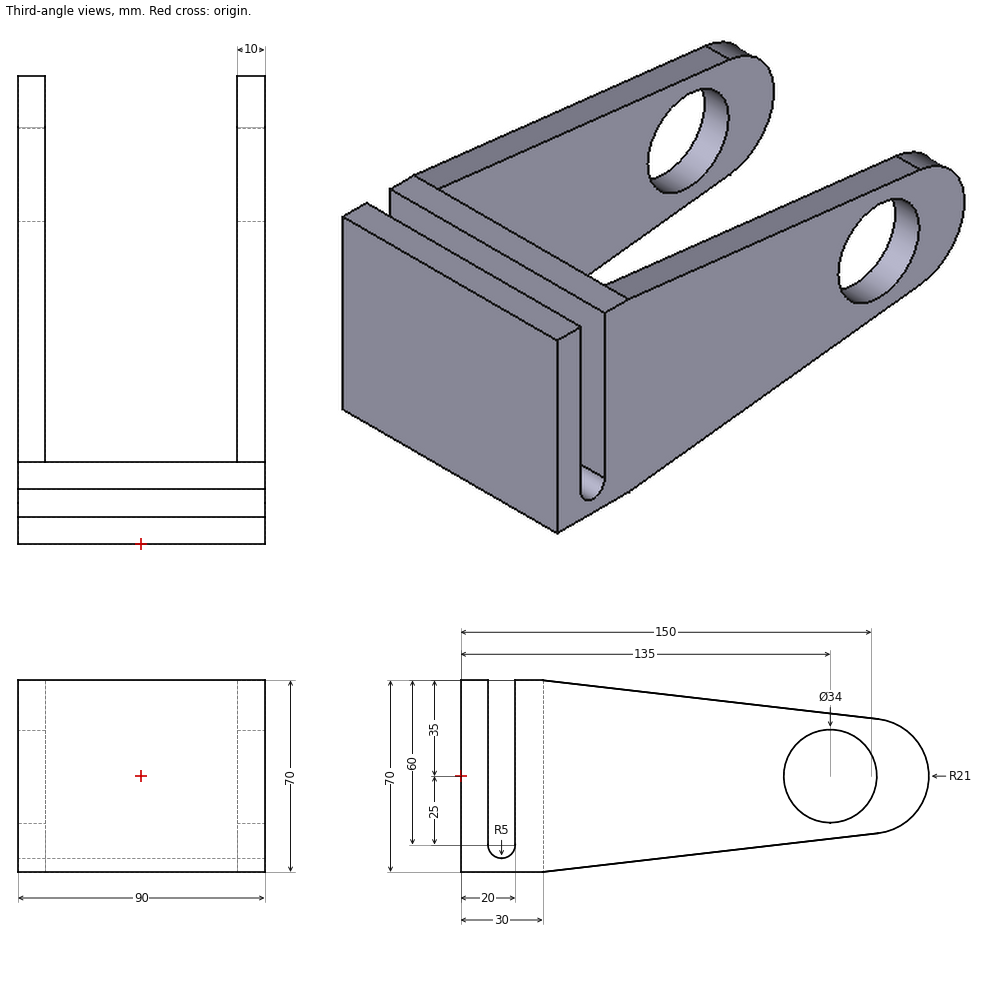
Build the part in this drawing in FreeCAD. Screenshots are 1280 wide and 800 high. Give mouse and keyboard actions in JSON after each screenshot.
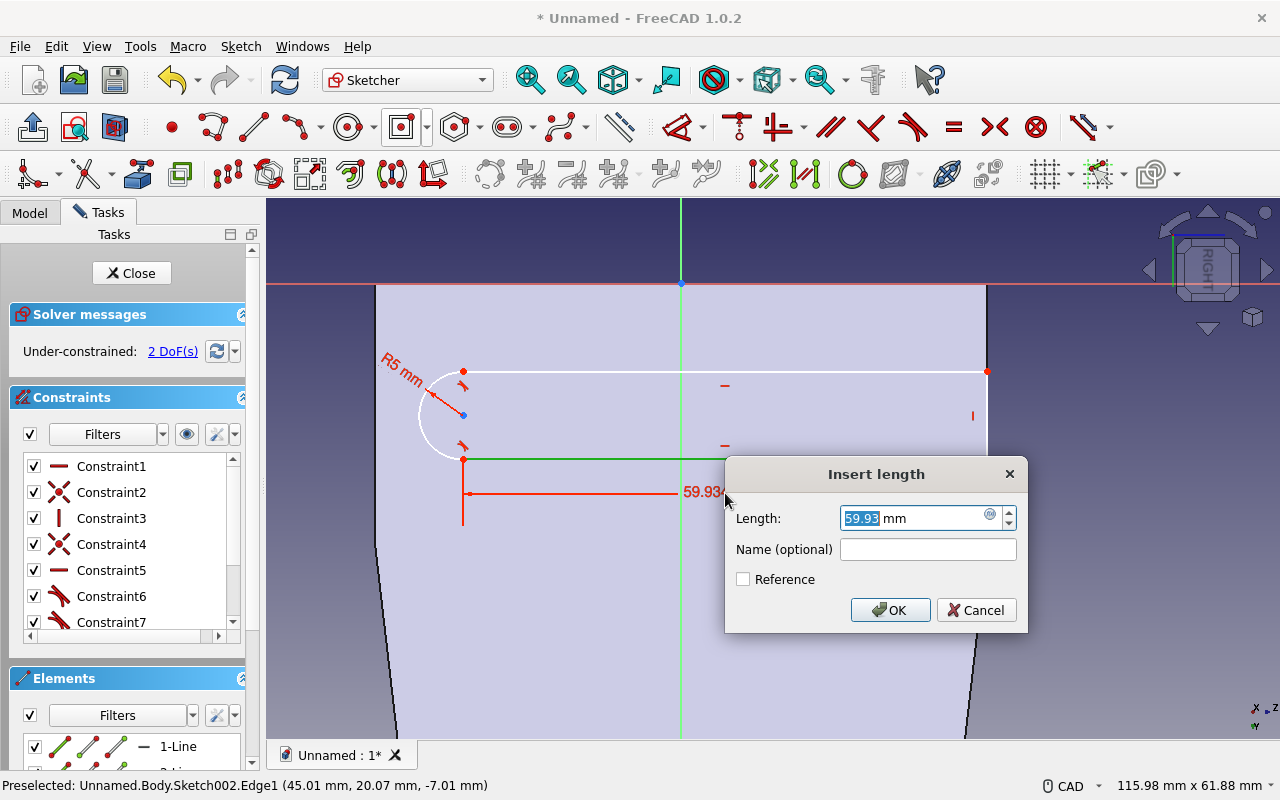
{"action": "type", "text": "60"}
{"action": "key", "text": "Return"}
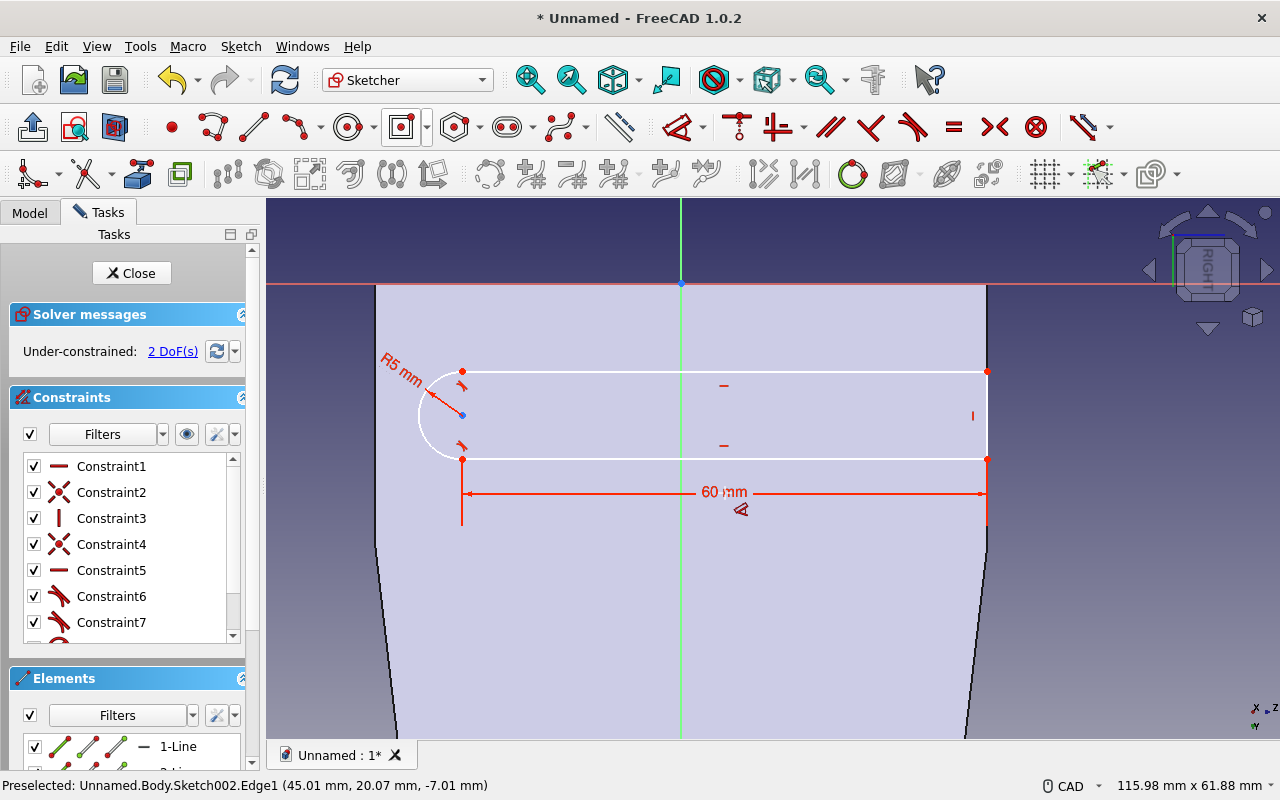
{"action": "left_click", "coordinate": [462, 459]}
{"action": "left_click", "coordinate": [572, 493]}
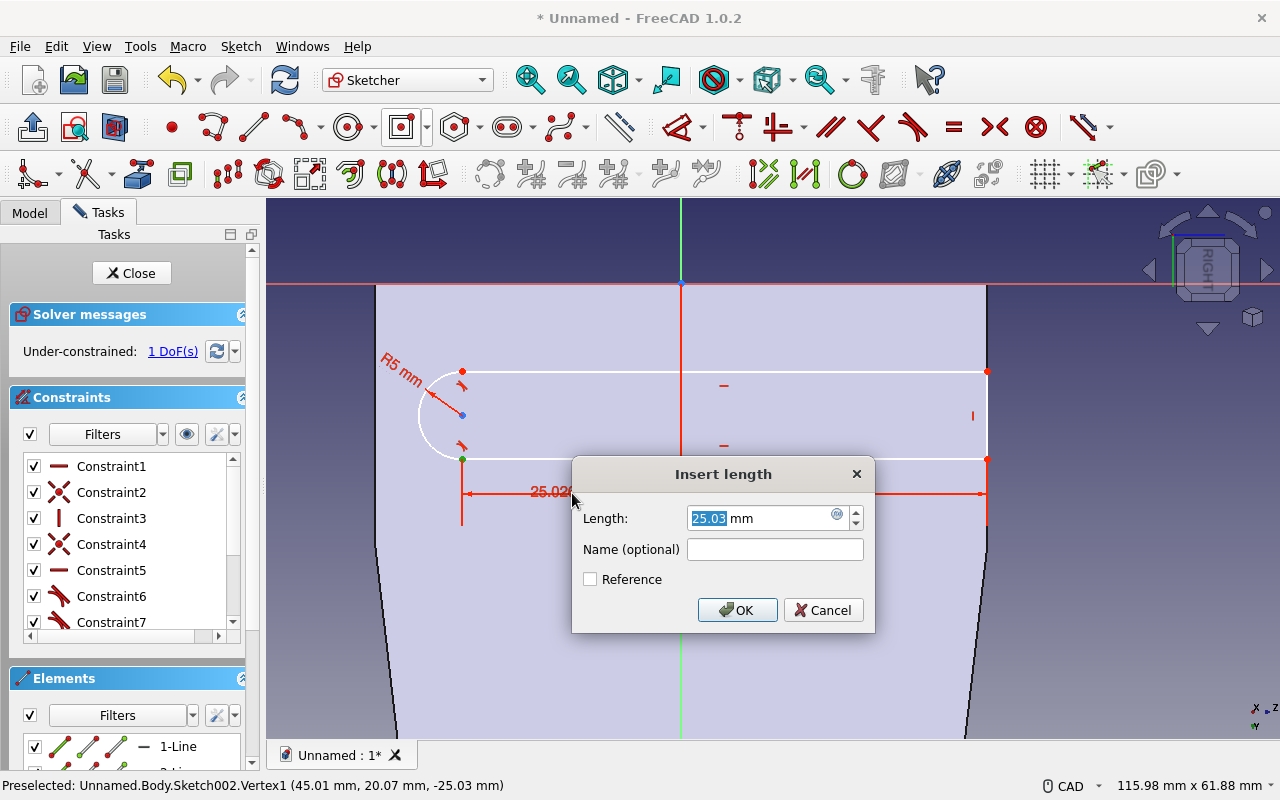
{"action": "type", "text": "25"}
{"action": "key", "text": "Return"}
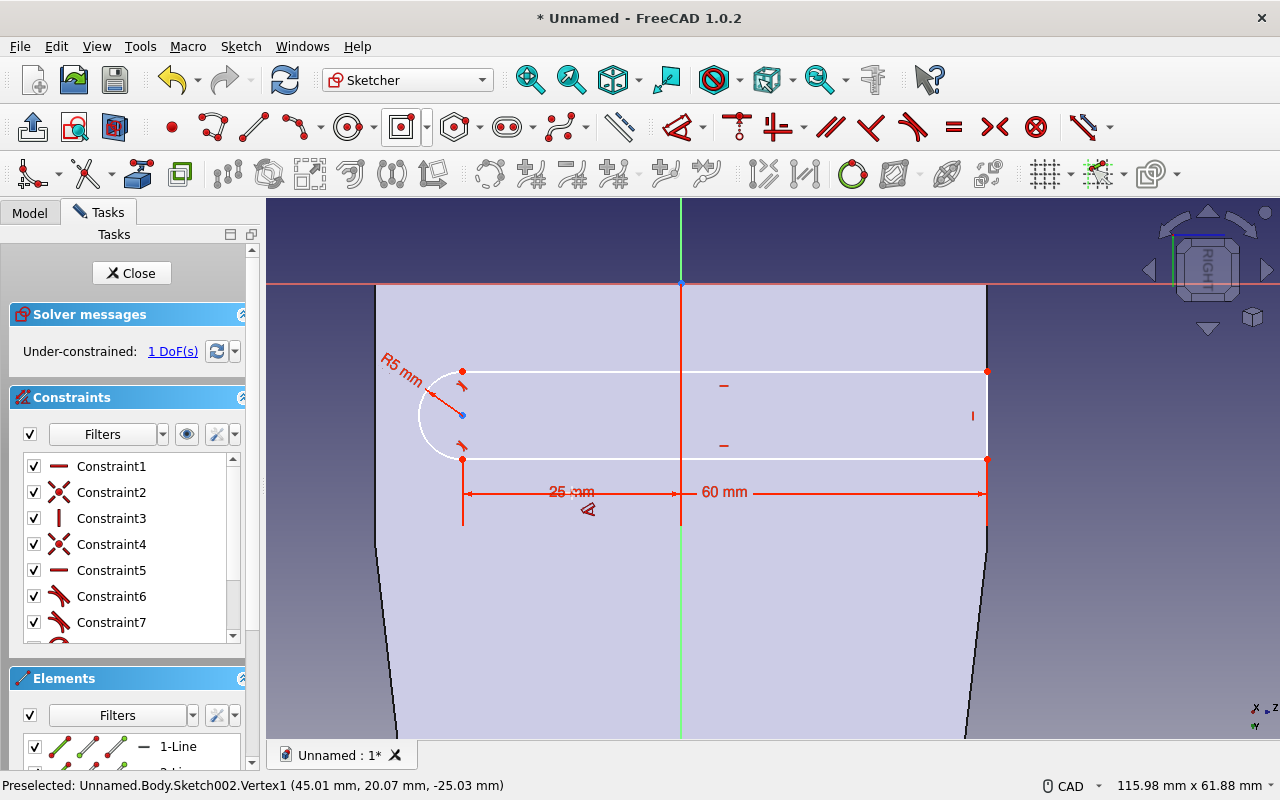
{"action": "left_click", "coordinate": [463, 459]}
{"action": "left_click", "coordinate": [429, 331]}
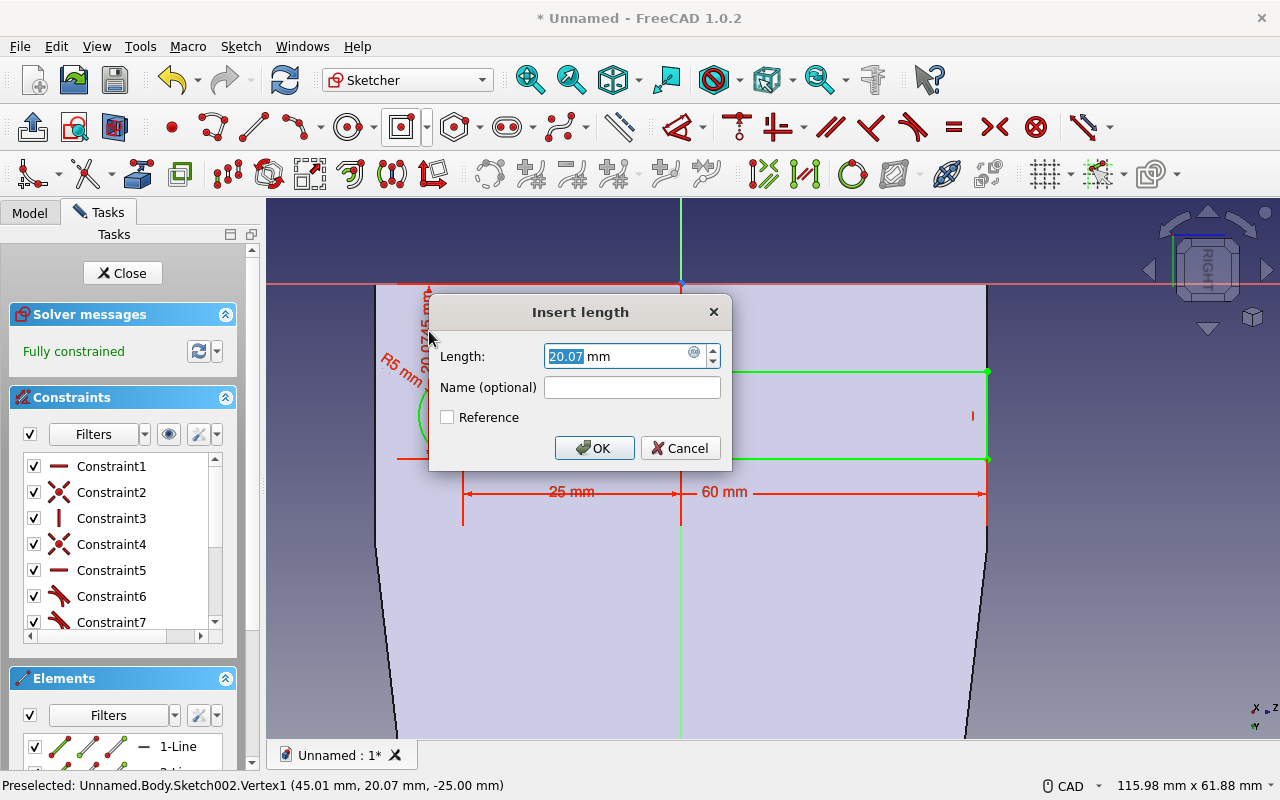
{"action": "type", "text": "20"}
{"action": "key", "text": "Return"}
{"action": "key", "text": "Escape"}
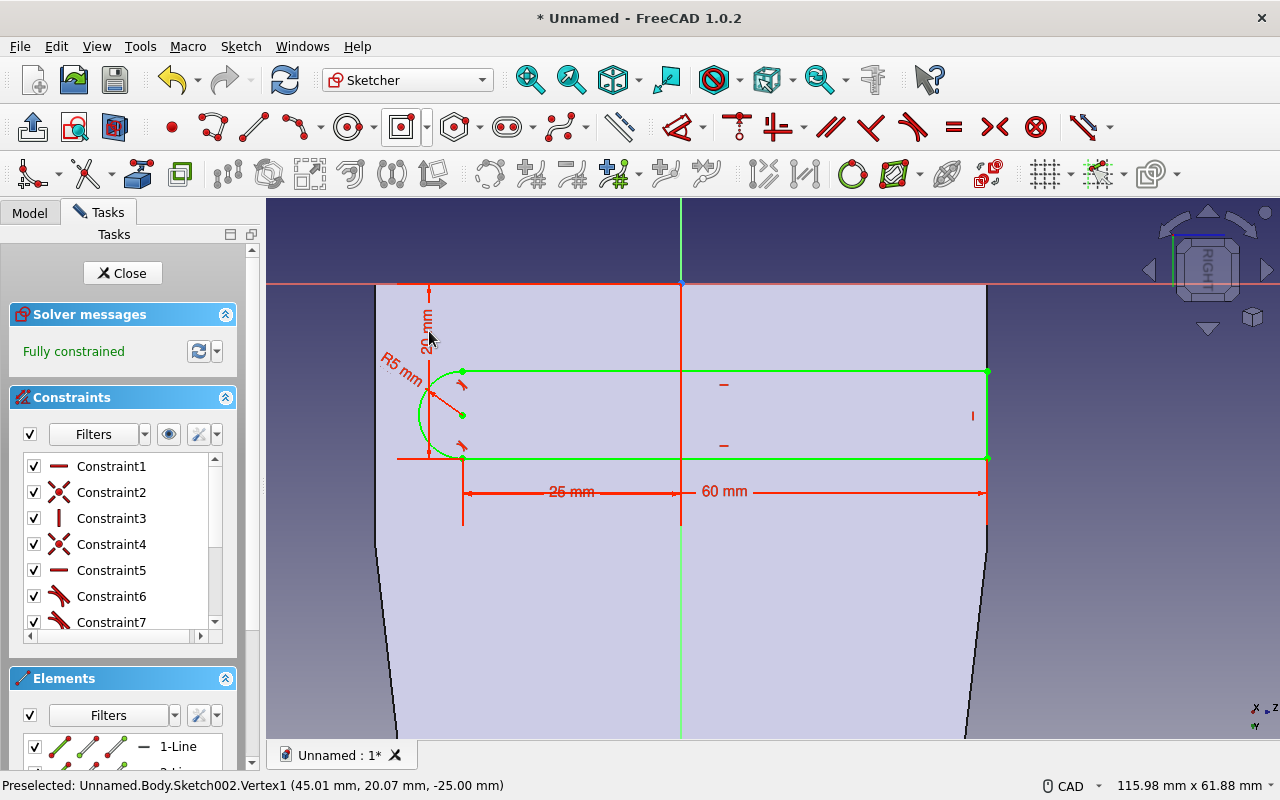
{"action": "left_click", "coordinate": [123, 273]}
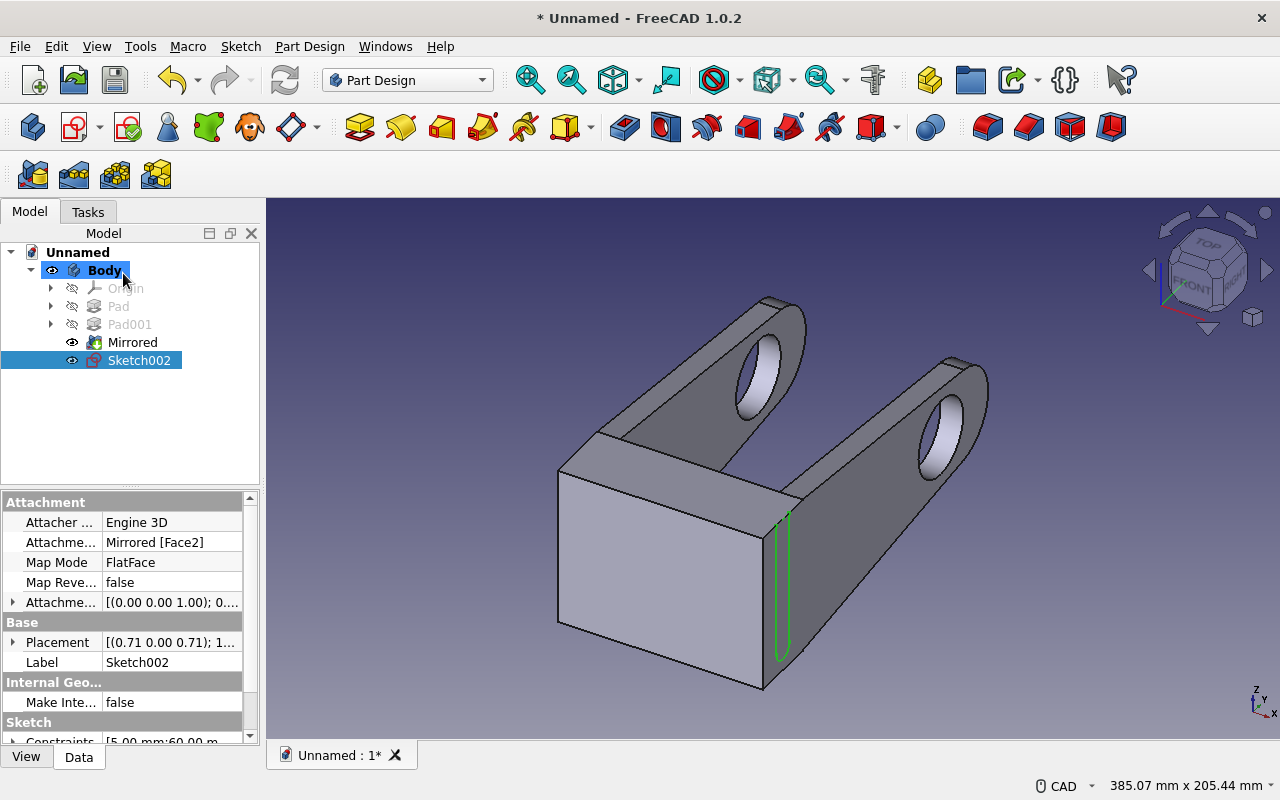
{"action": "left_click", "coordinate": [625, 128]}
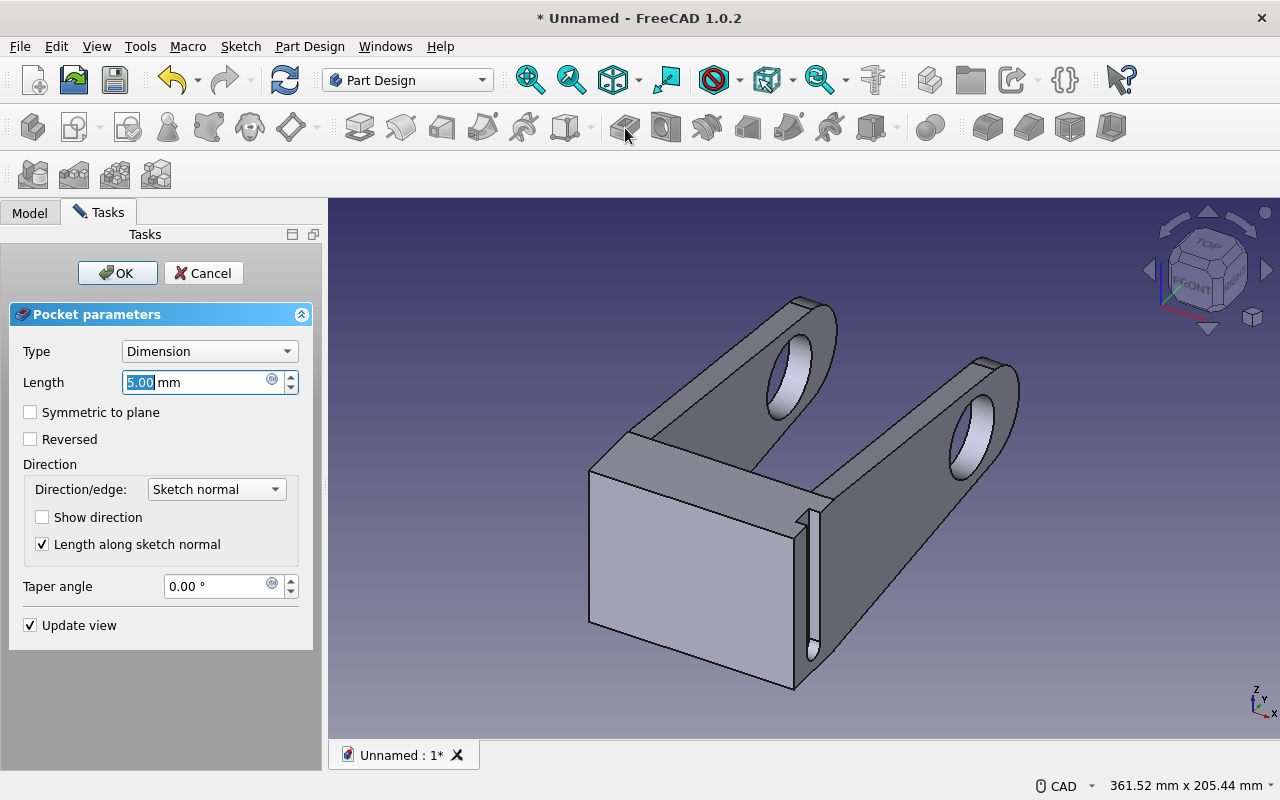
{"action": "left_click", "coordinate": [210, 352]}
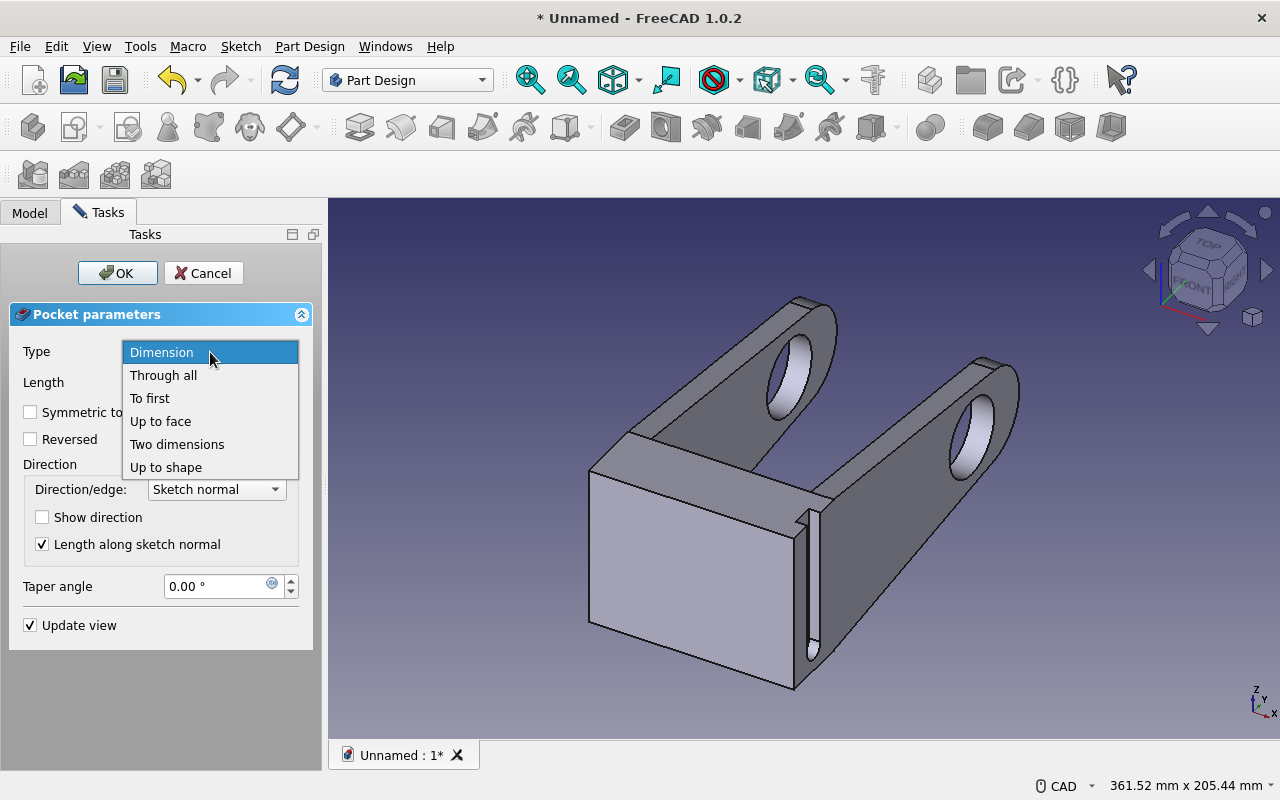
{"action": "left_click", "coordinate": [208, 376]}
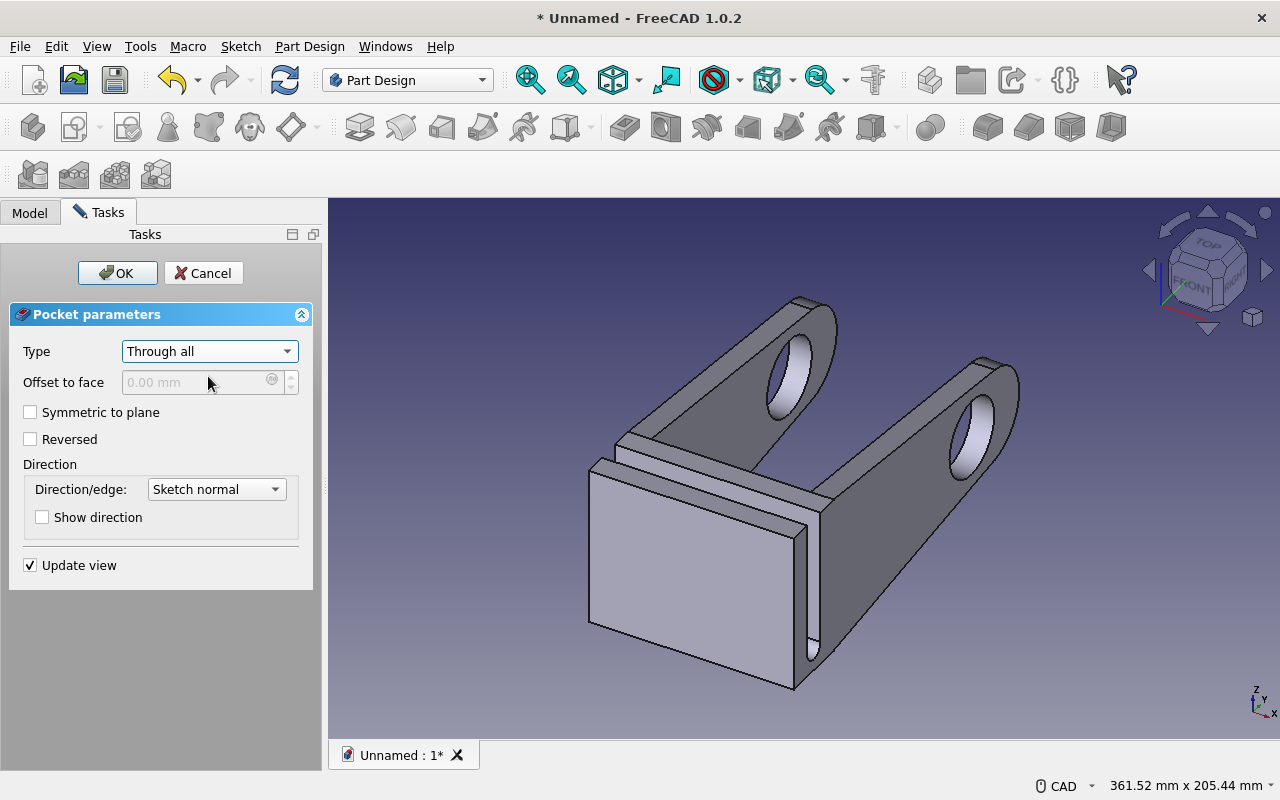
{"action": "left_click", "coordinate": [118, 273]}